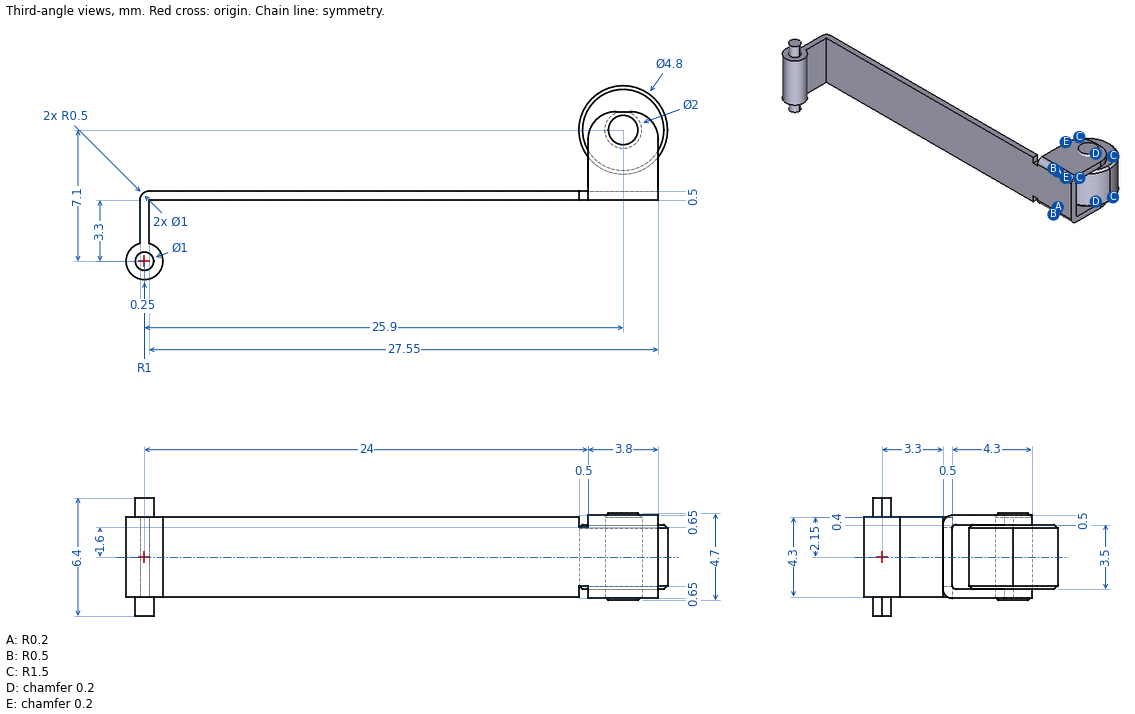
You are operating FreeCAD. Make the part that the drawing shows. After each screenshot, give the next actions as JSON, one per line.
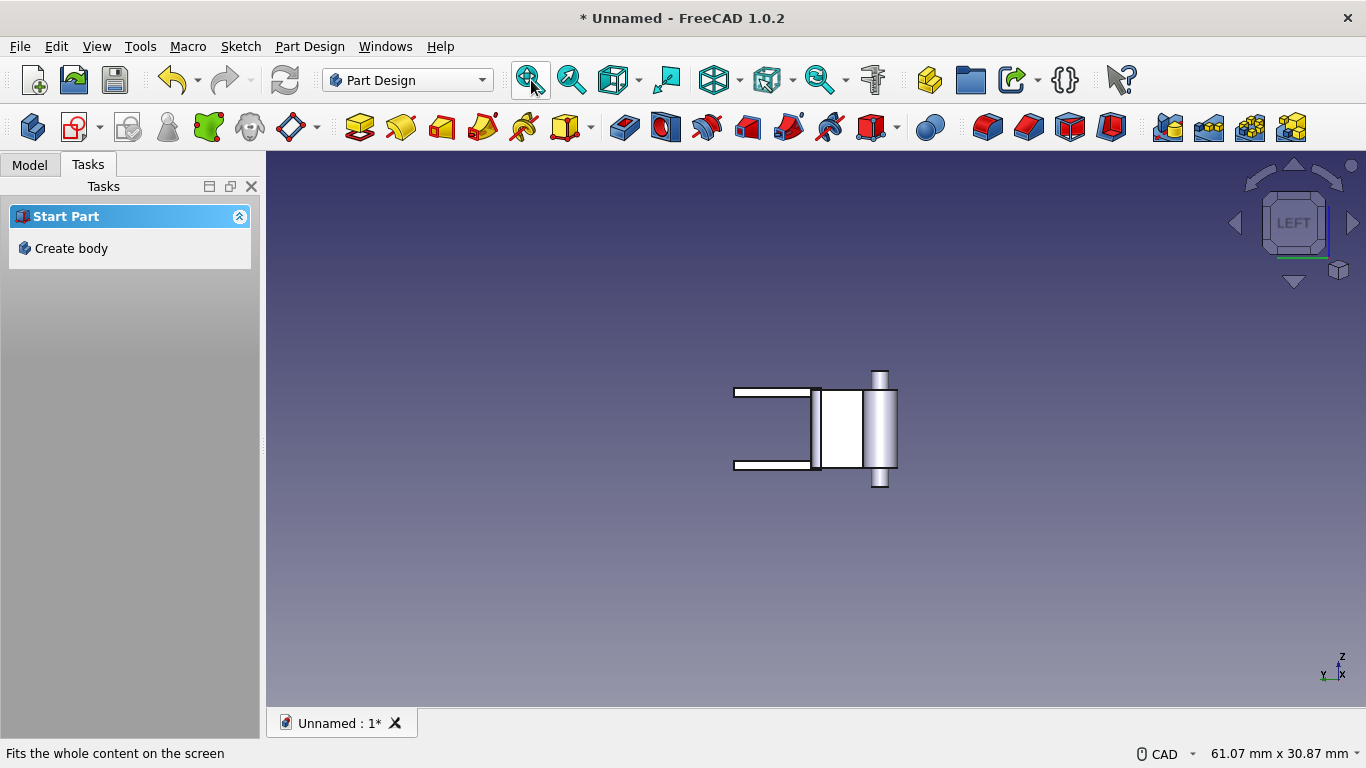
{"action": "key", "text": "0"}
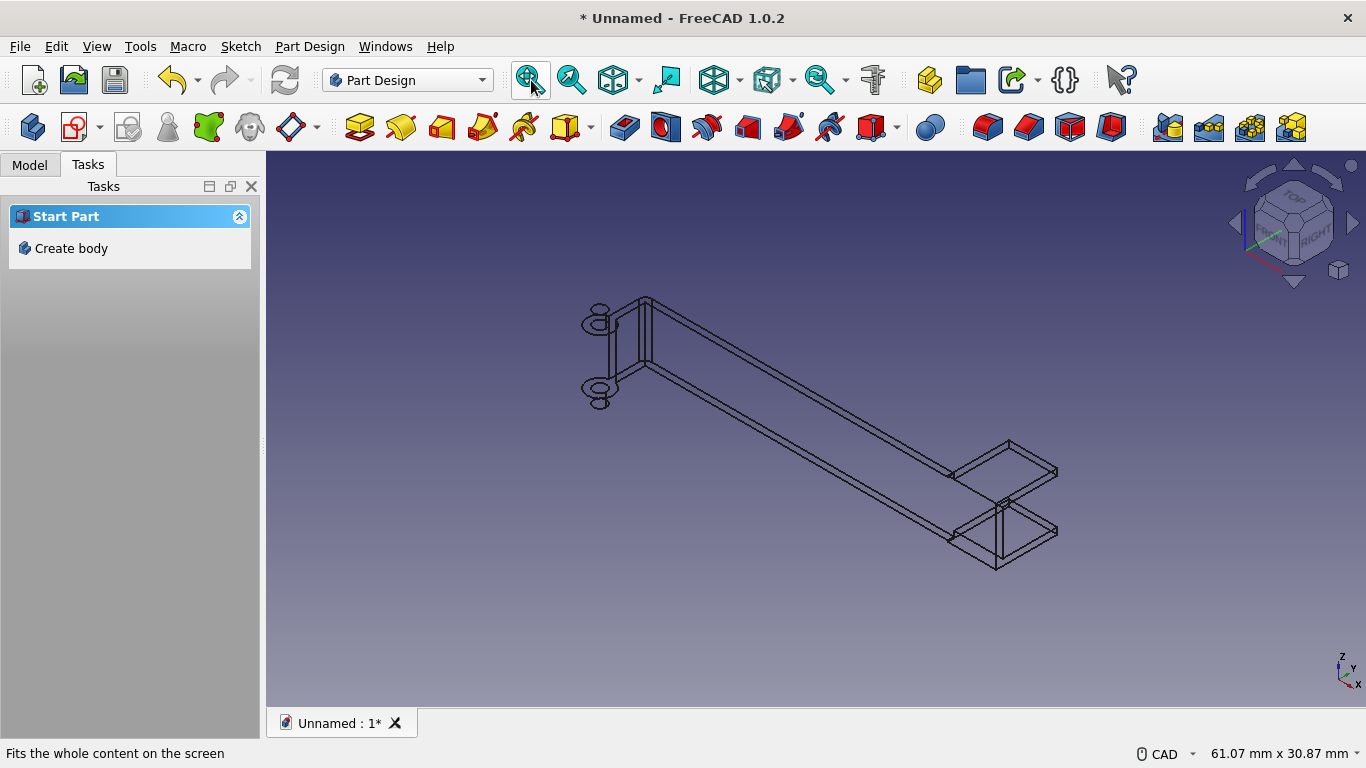
{"action": "left_click", "coordinate": [978, 544]}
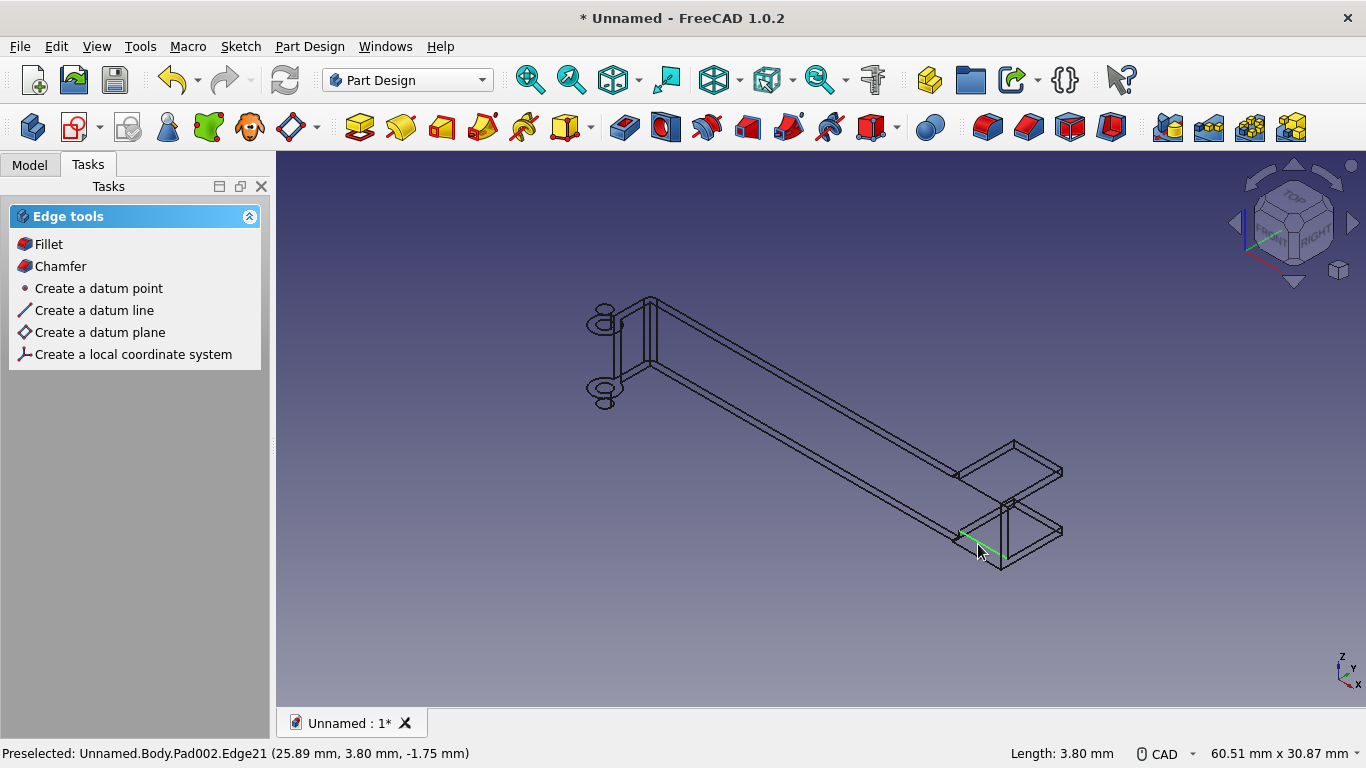
{"action": "scroll", "coordinate": [983, 492], "scroll_direction": "up", "scroll_amount": 6}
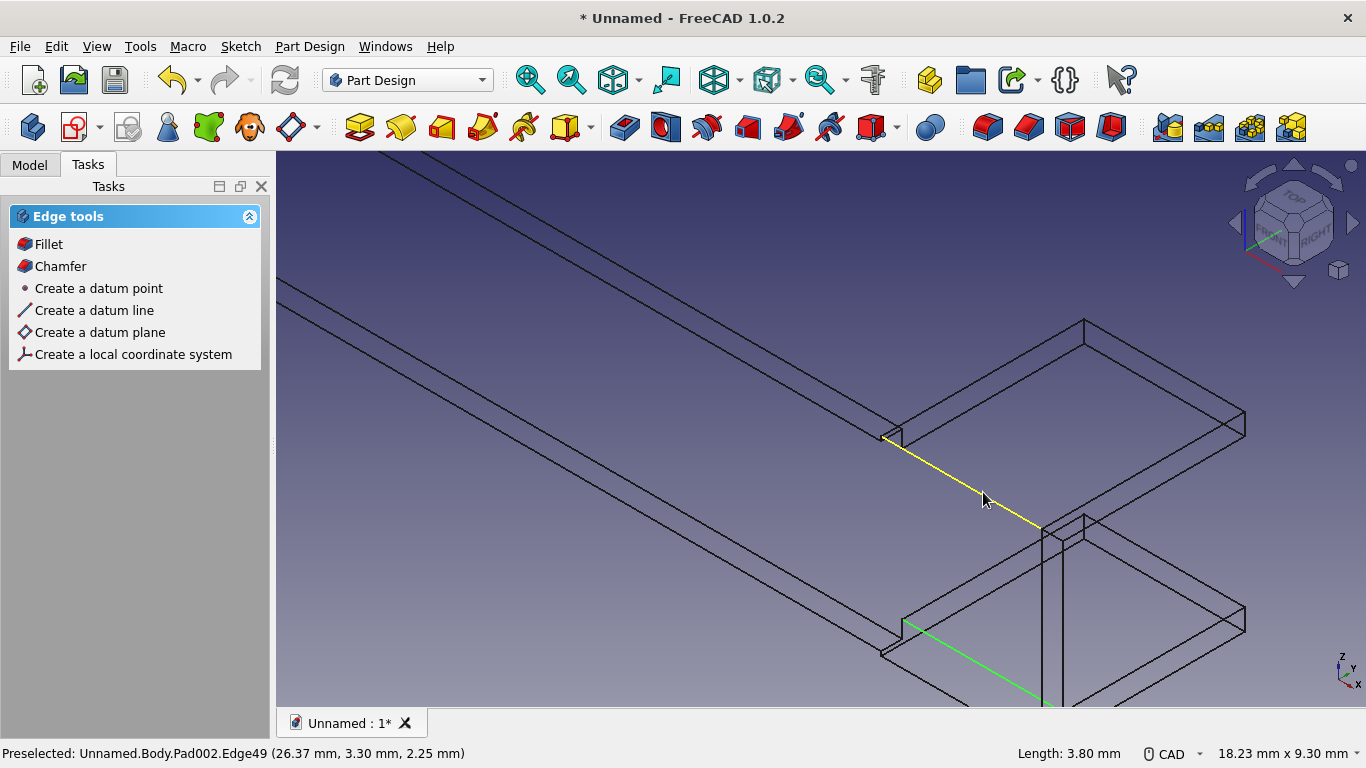
{"action": "key", "text": "v f"}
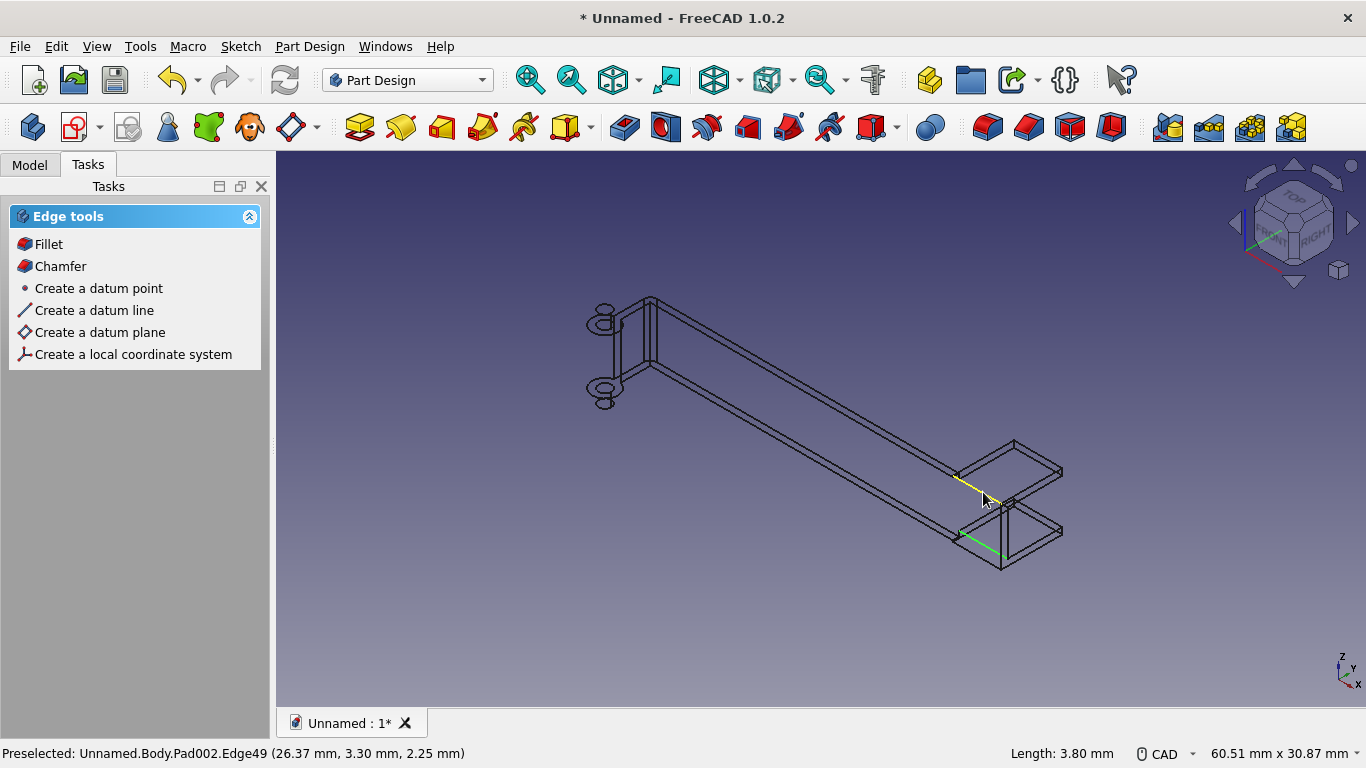
{"action": "key", "text": "2"}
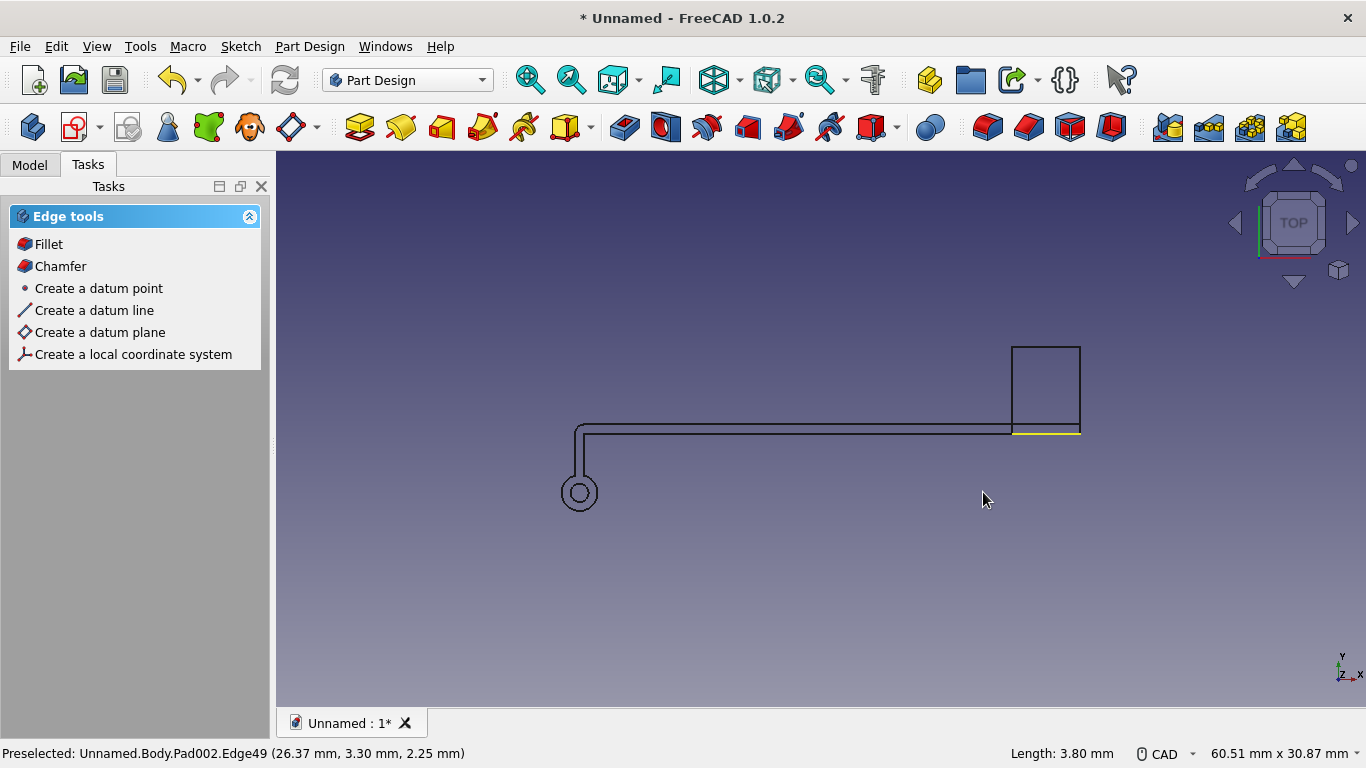
{"action": "left_click", "coordinate": [1046, 423], "text": "ctrl"}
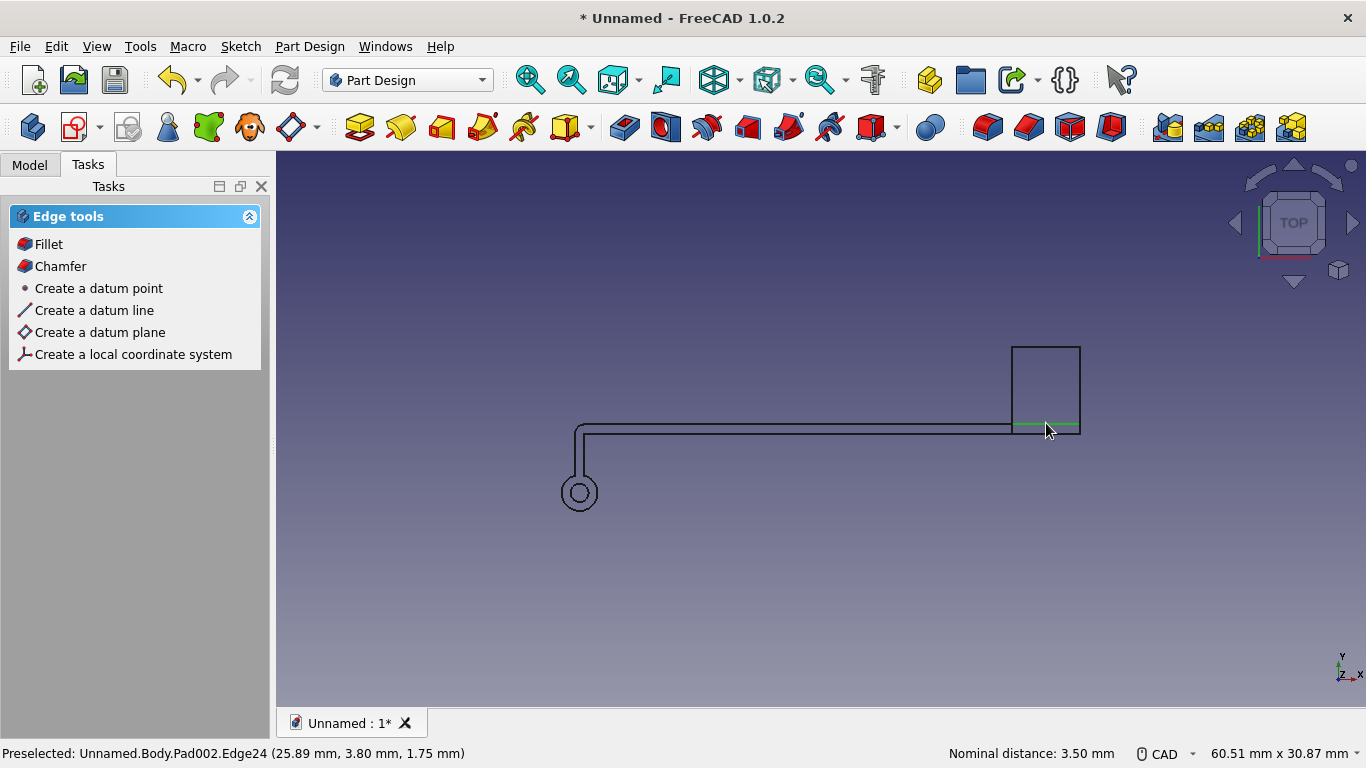
{"action": "key", "text": "v 1"}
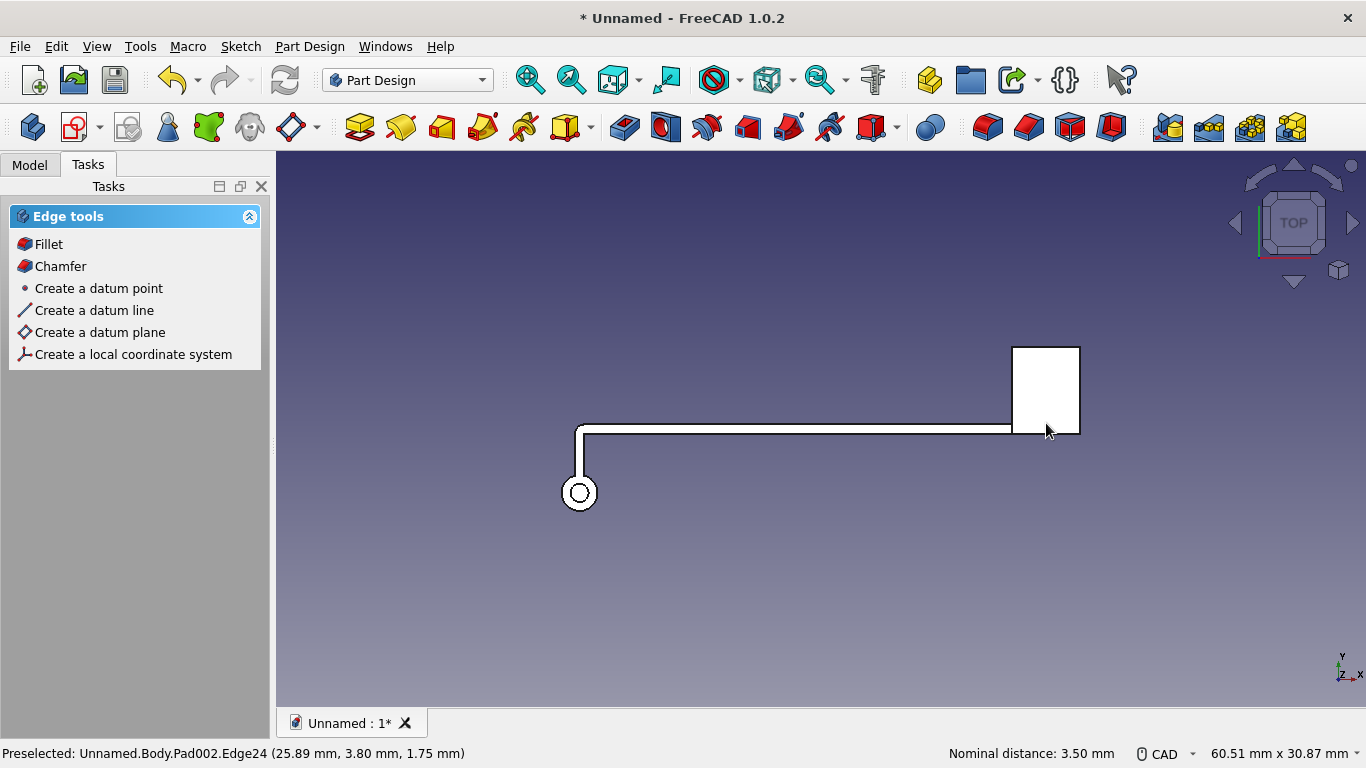
{"action": "left_click", "coordinate": [988, 128]}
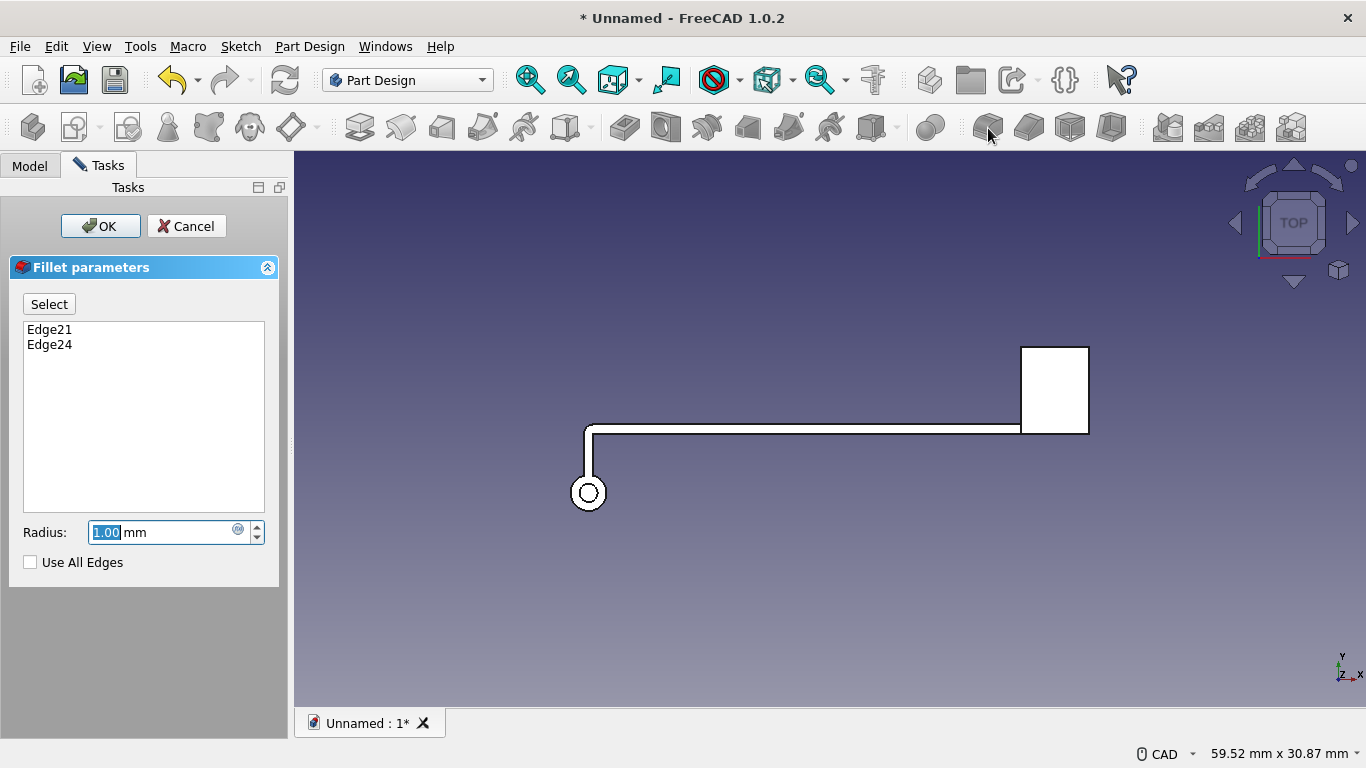
{"action": "type", "text": "0.2"}
{"action": "key", "text": "Tab"}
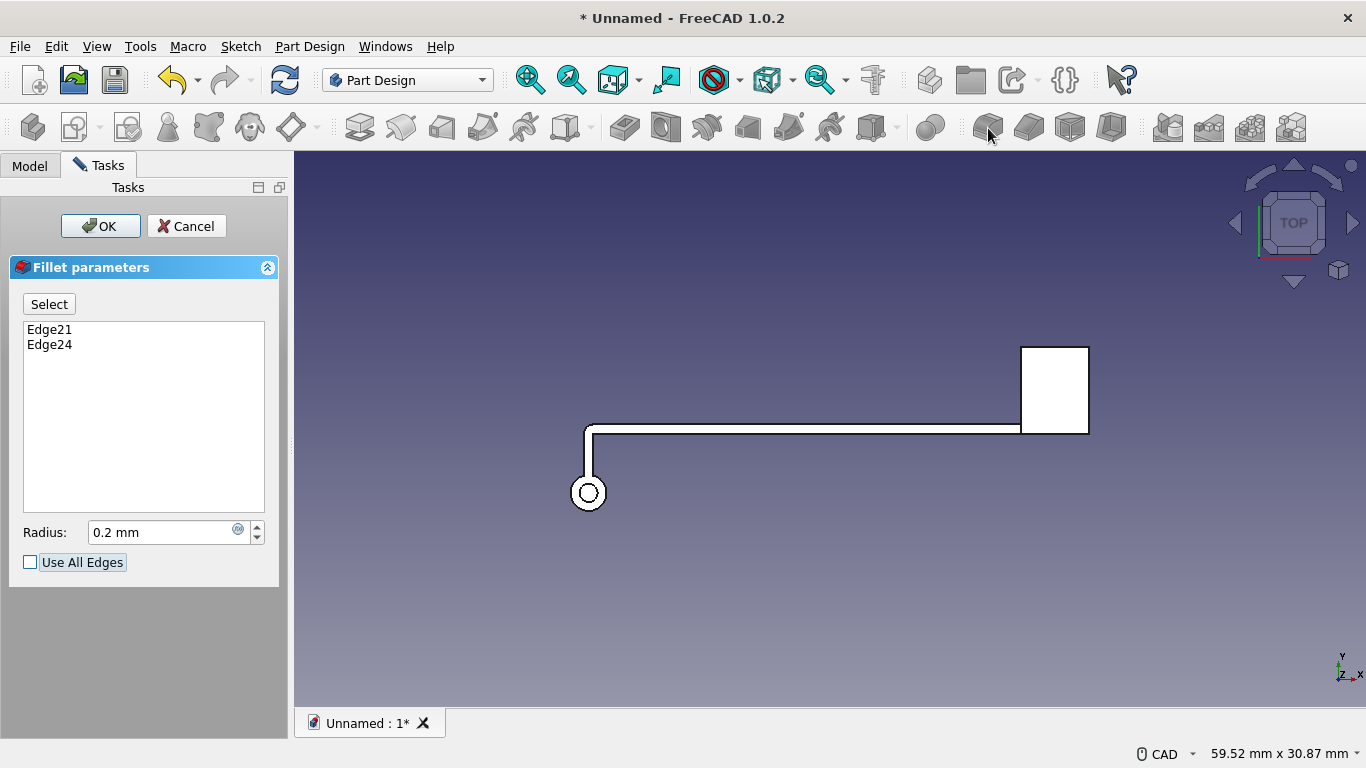
{"action": "left_click", "coordinate": [101, 226]}